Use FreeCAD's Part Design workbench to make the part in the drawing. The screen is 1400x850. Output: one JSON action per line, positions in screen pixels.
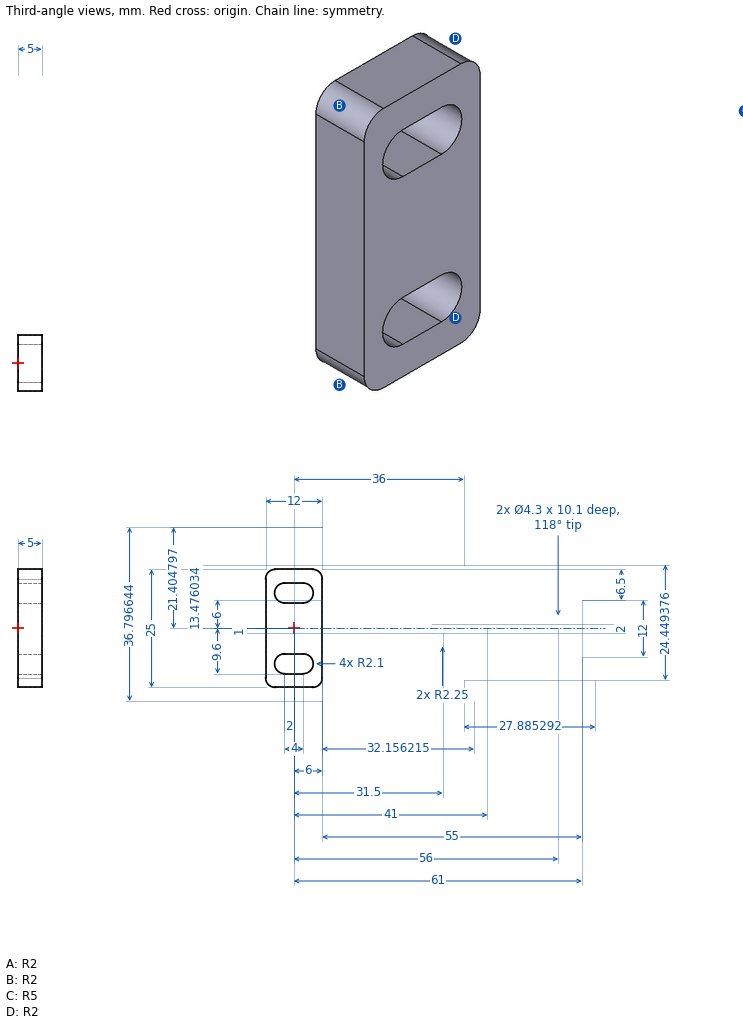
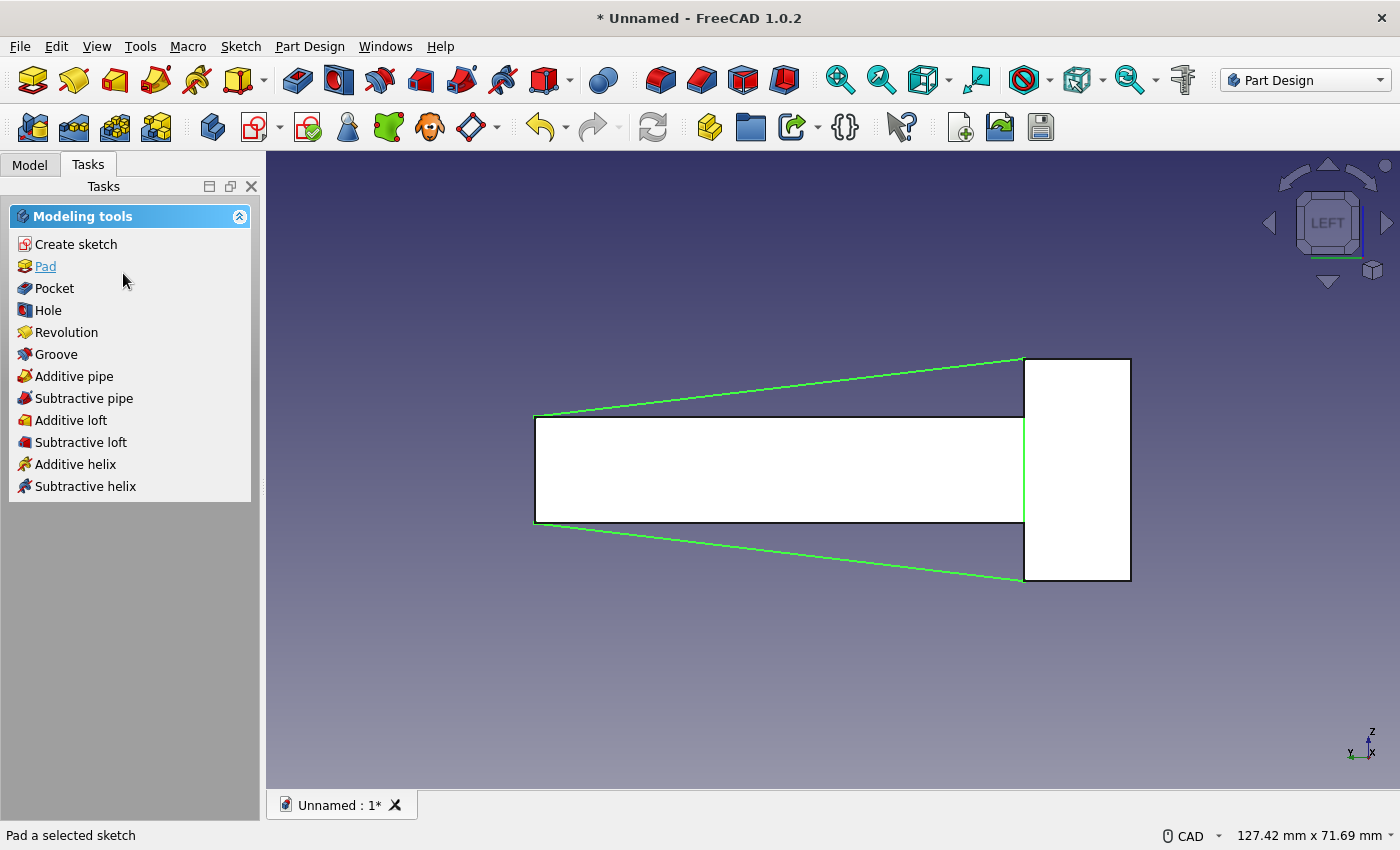
{"action": "left_click", "coordinate": [33, 80]}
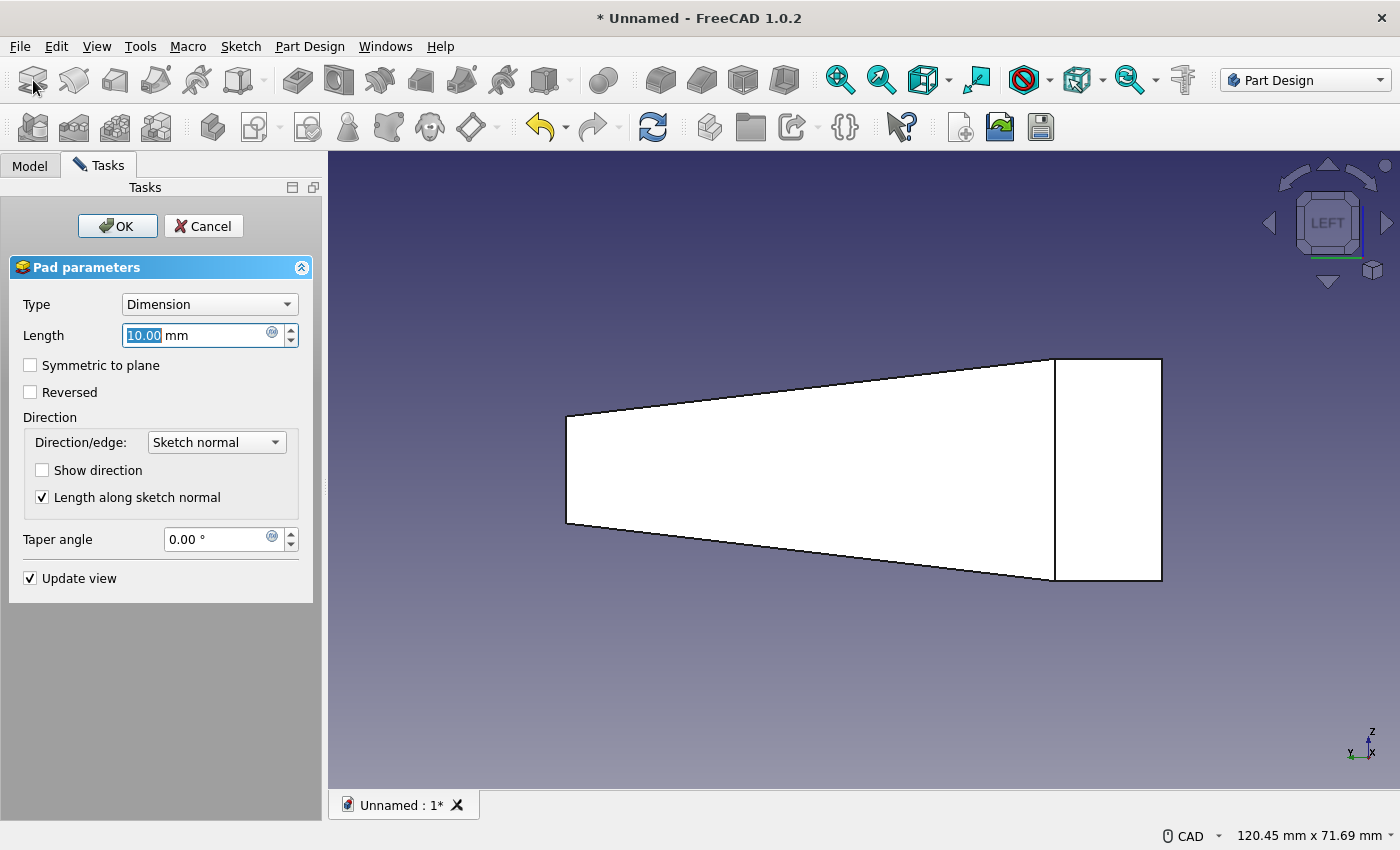
{"action": "type", "text": "5"}
{"action": "key", "text": "Tab"}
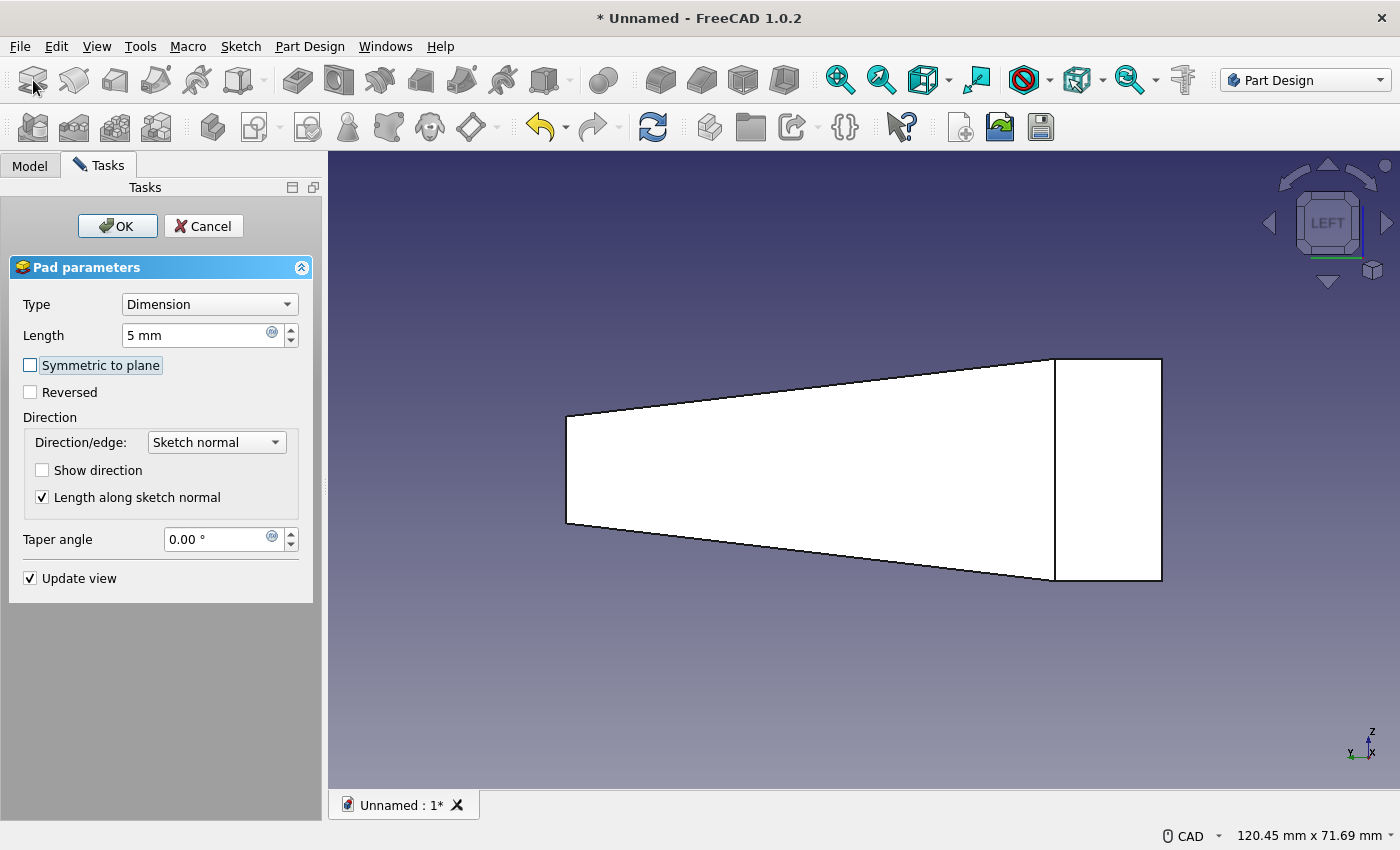
{"action": "left_click", "coordinate": [31, 392]}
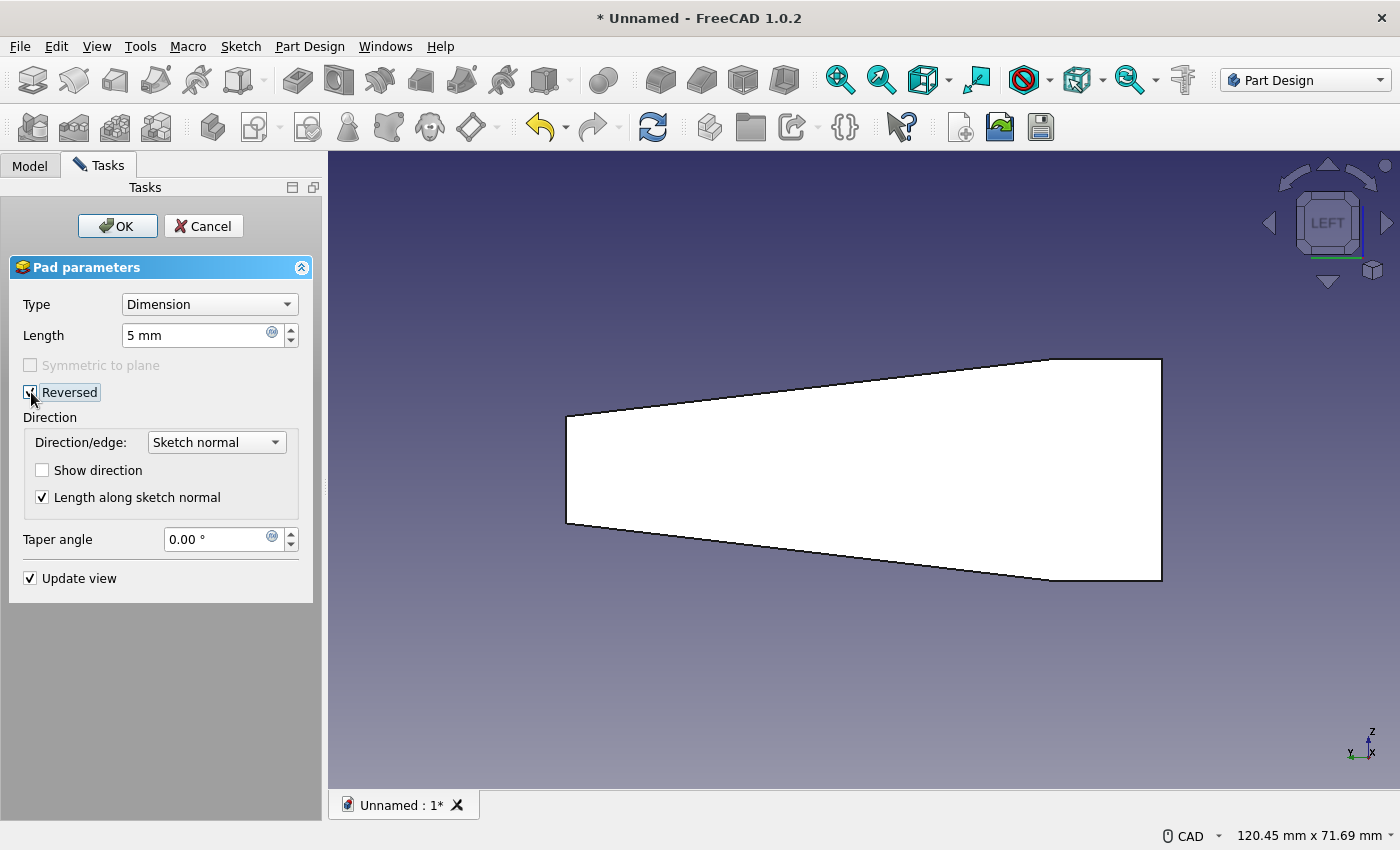
{"action": "left_click", "coordinate": [118, 226]}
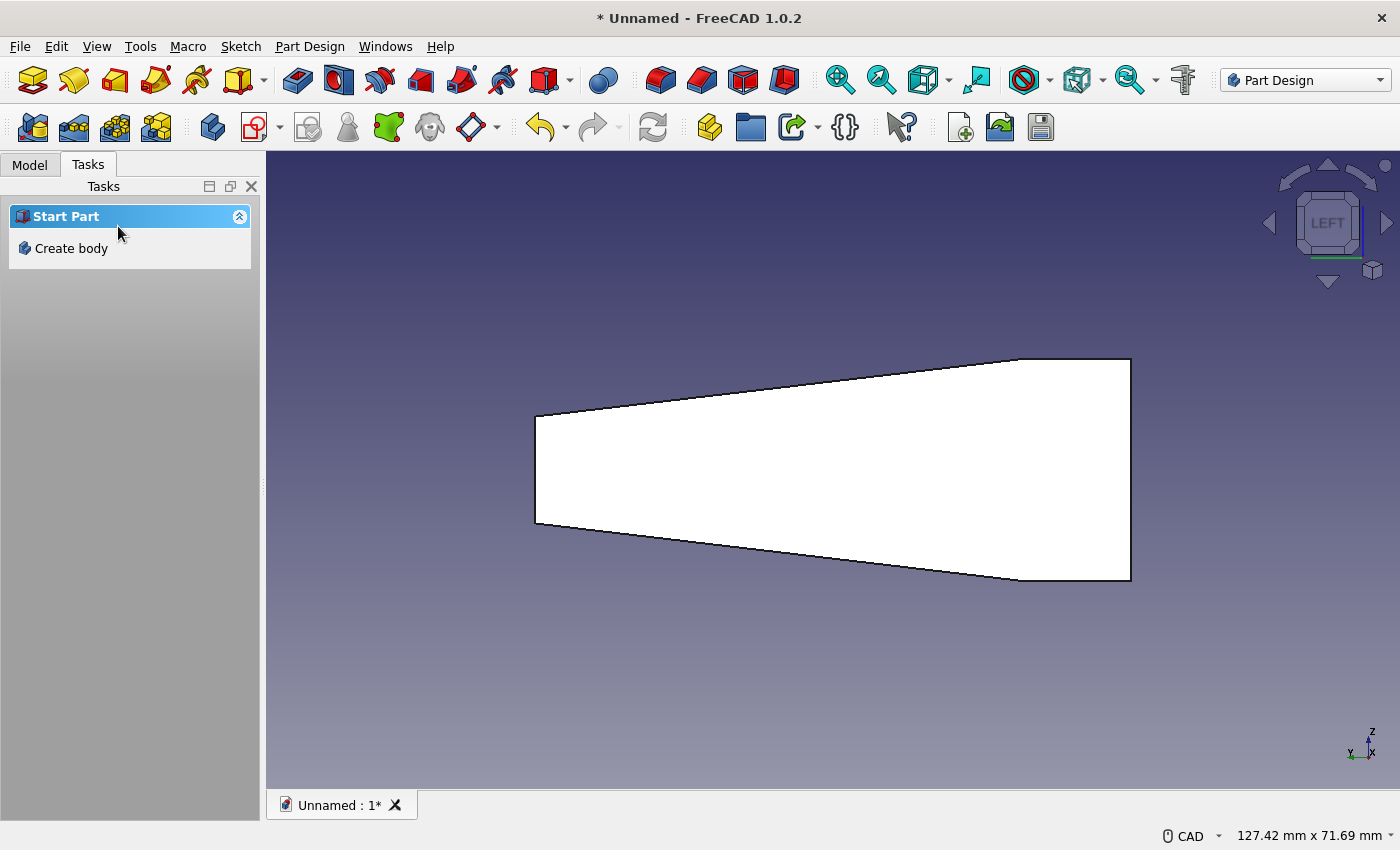
{"action": "key", "text": "0"}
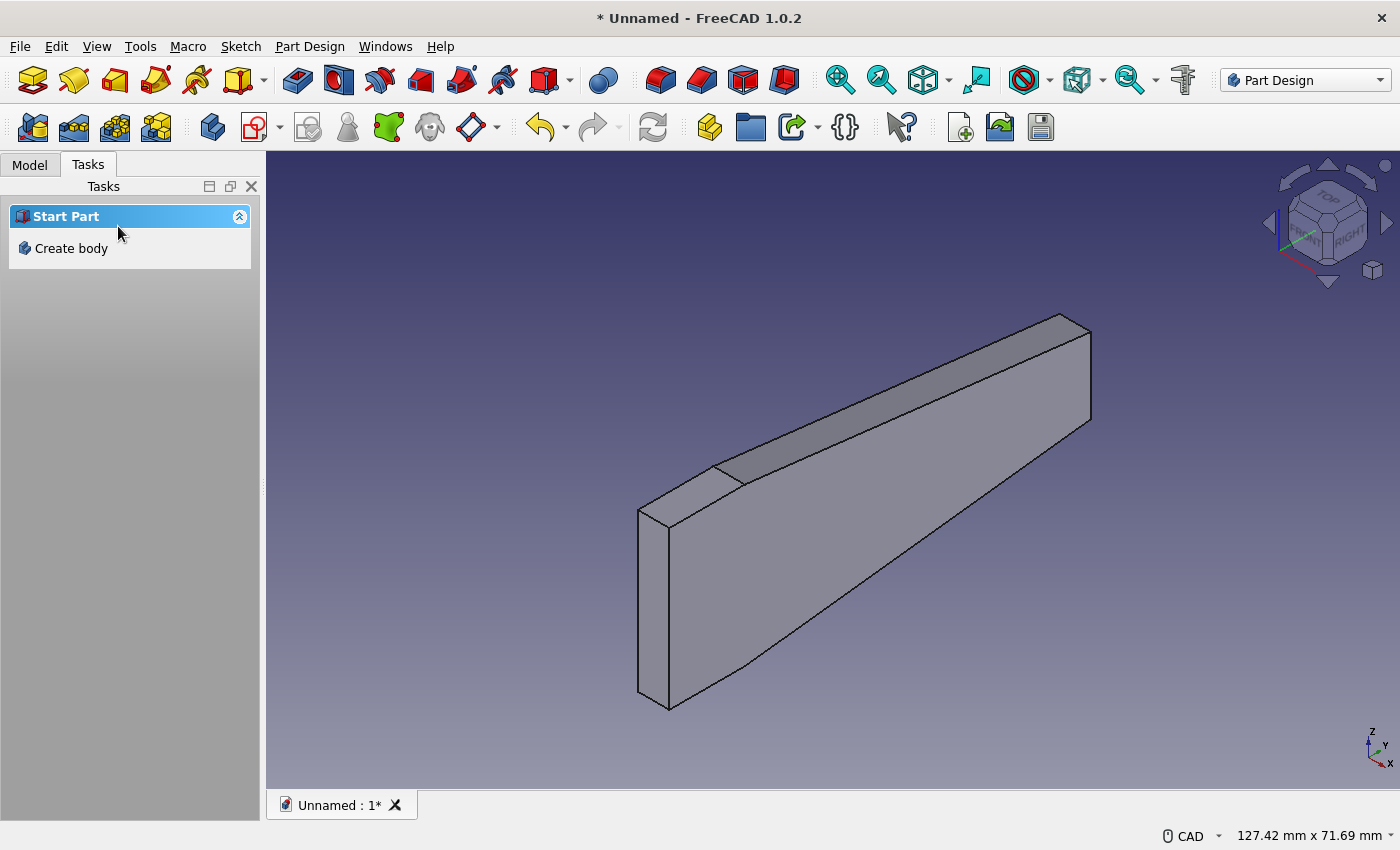
{"action": "key", "text": "2"}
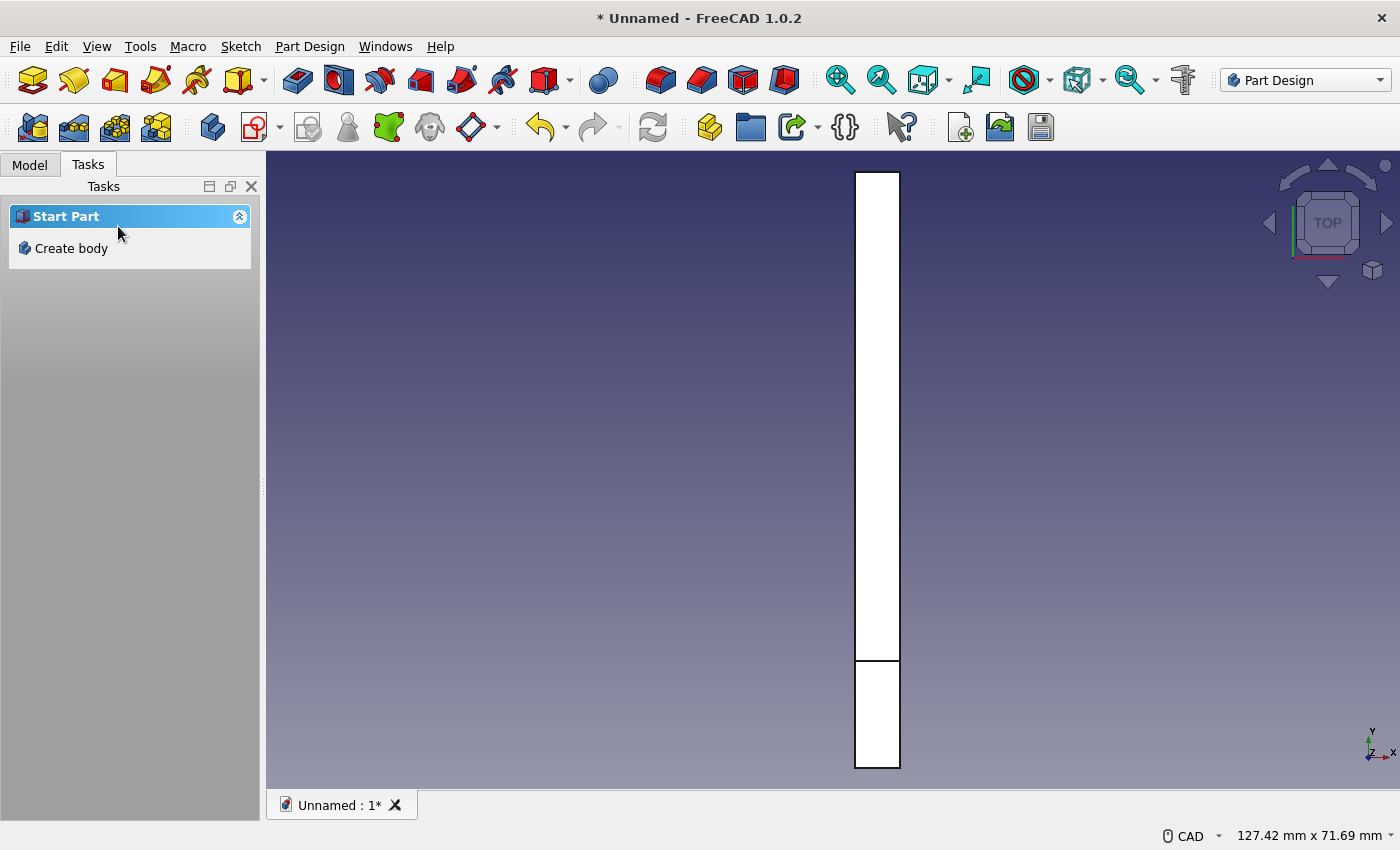
{"action": "key", "text": "1"}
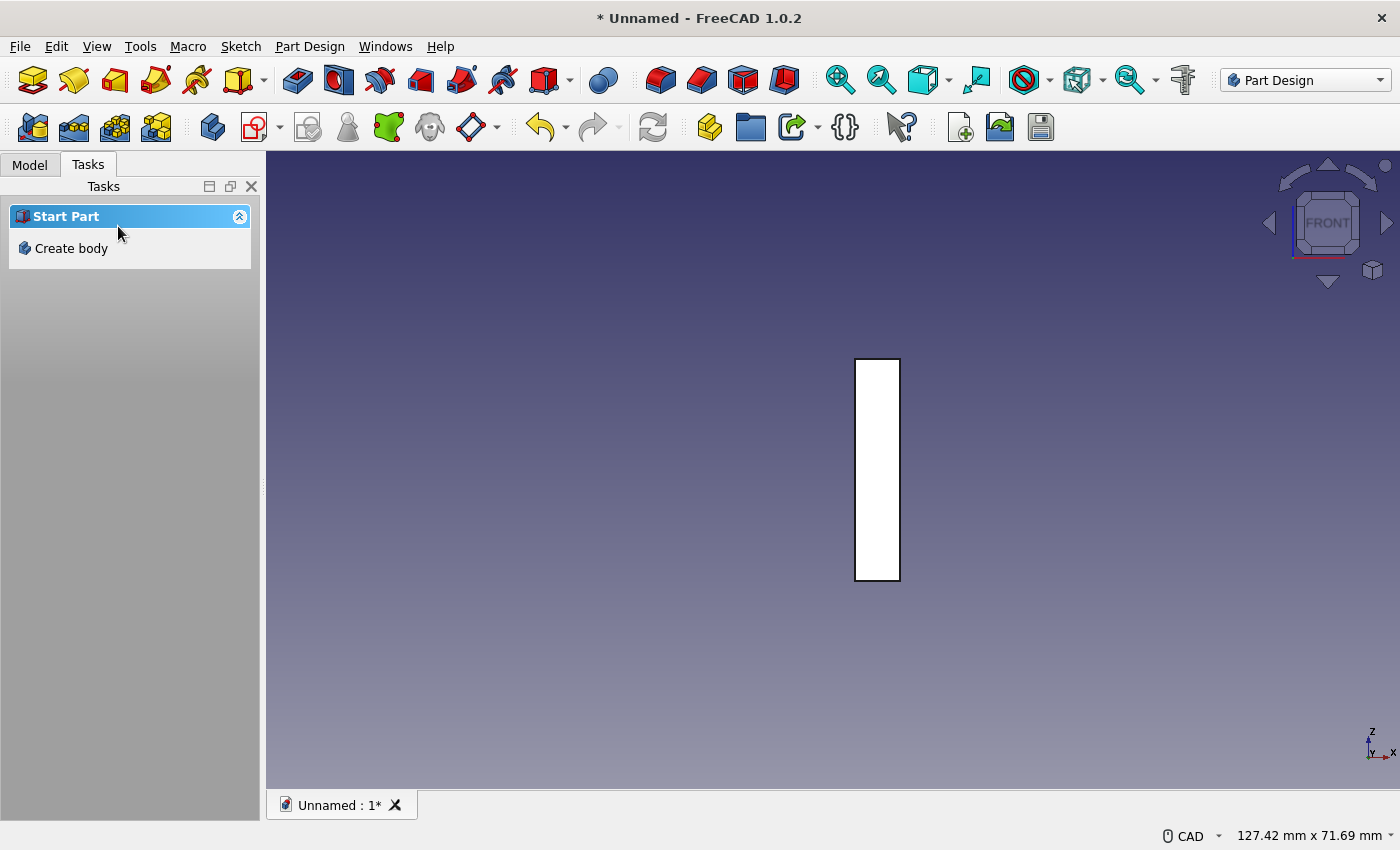
{"action": "left_click", "coordinate": [841, 80]}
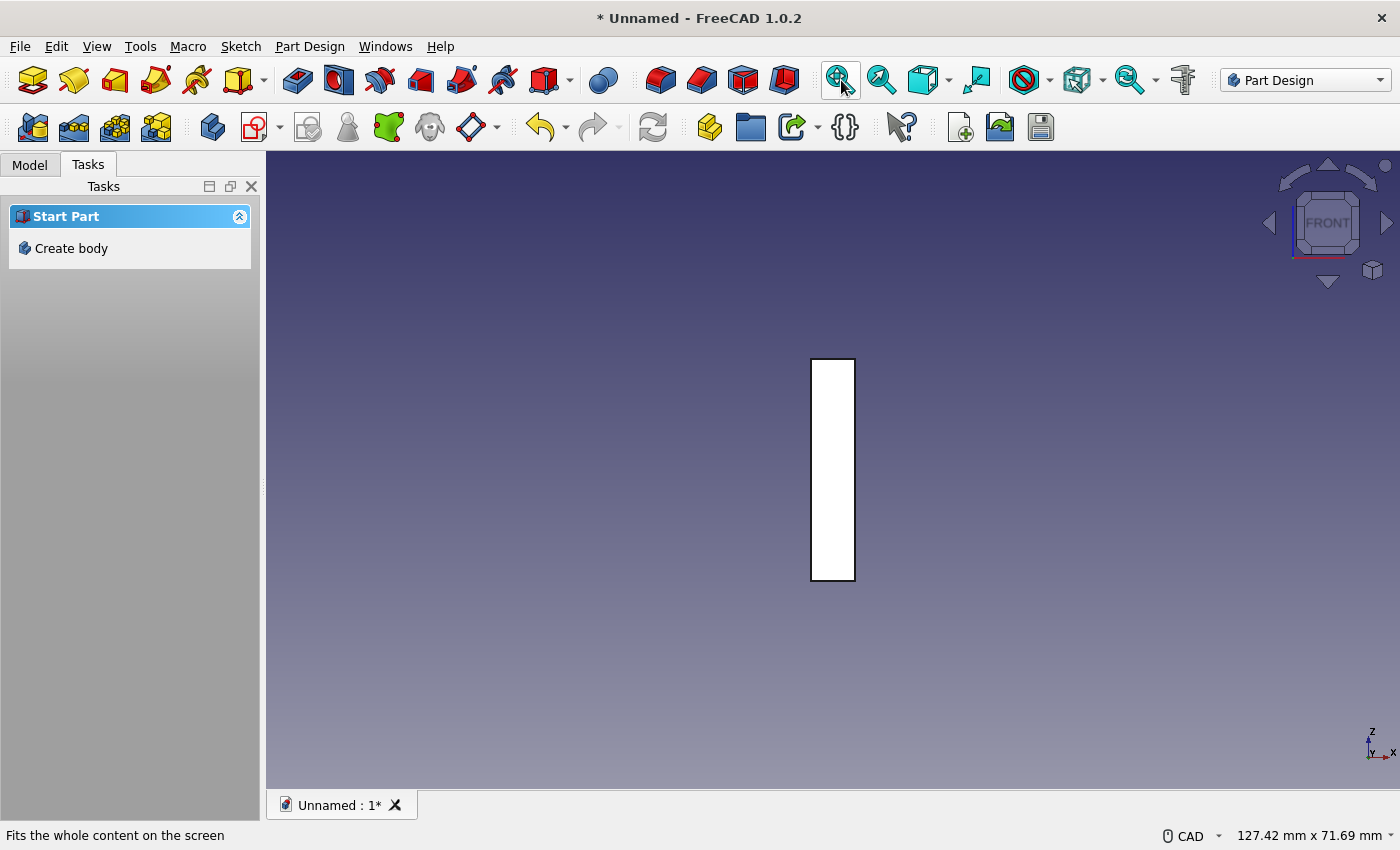
{"action": "key", "text": "3"}